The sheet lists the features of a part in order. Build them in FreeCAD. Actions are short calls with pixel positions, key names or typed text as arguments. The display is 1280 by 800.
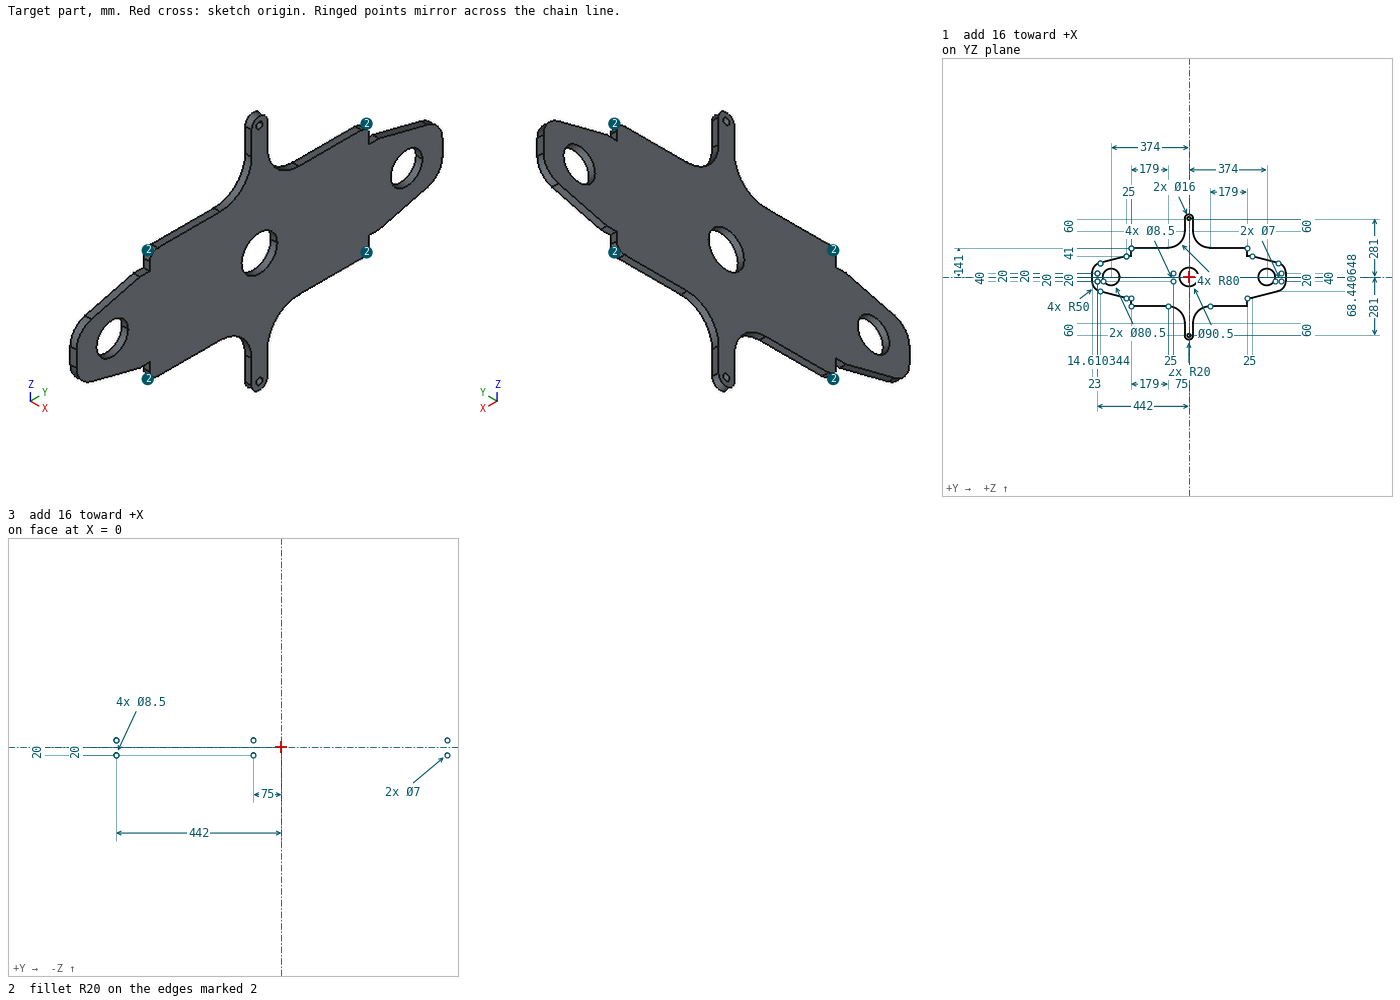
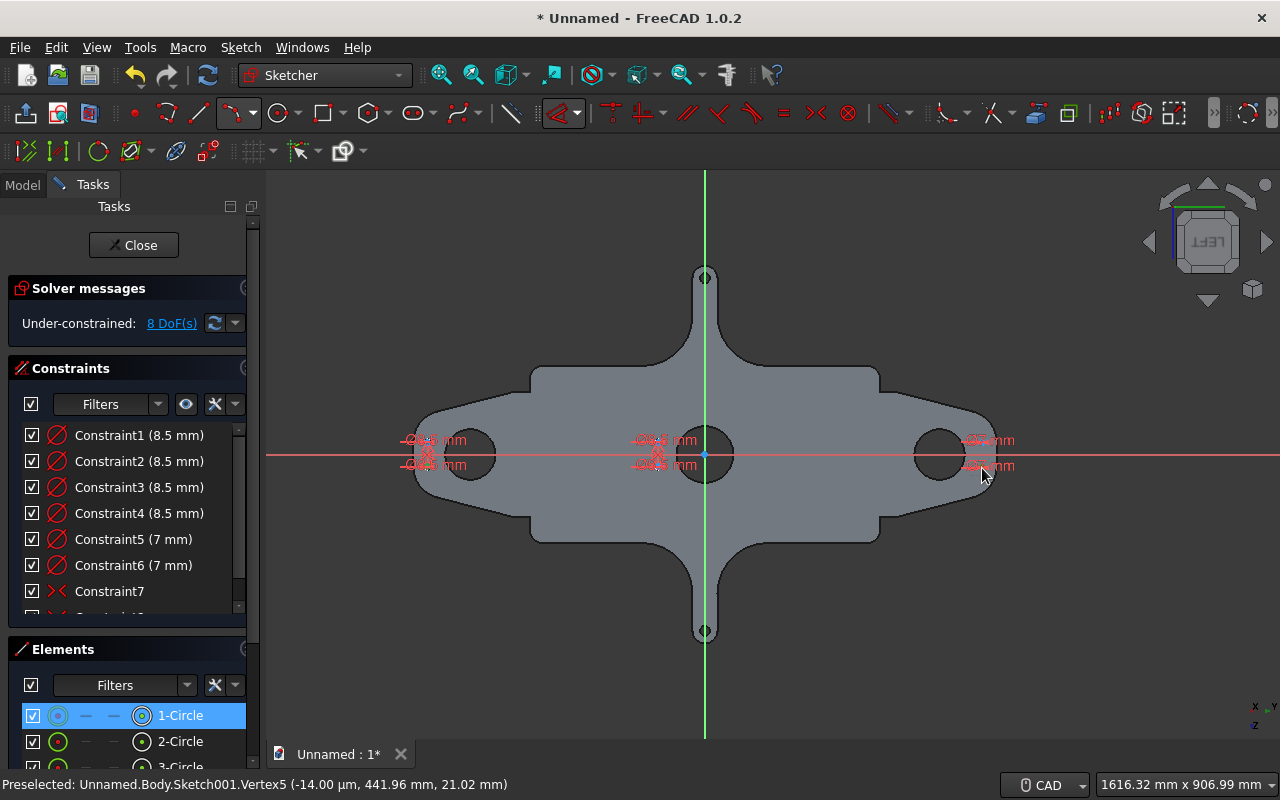
click(705, 674)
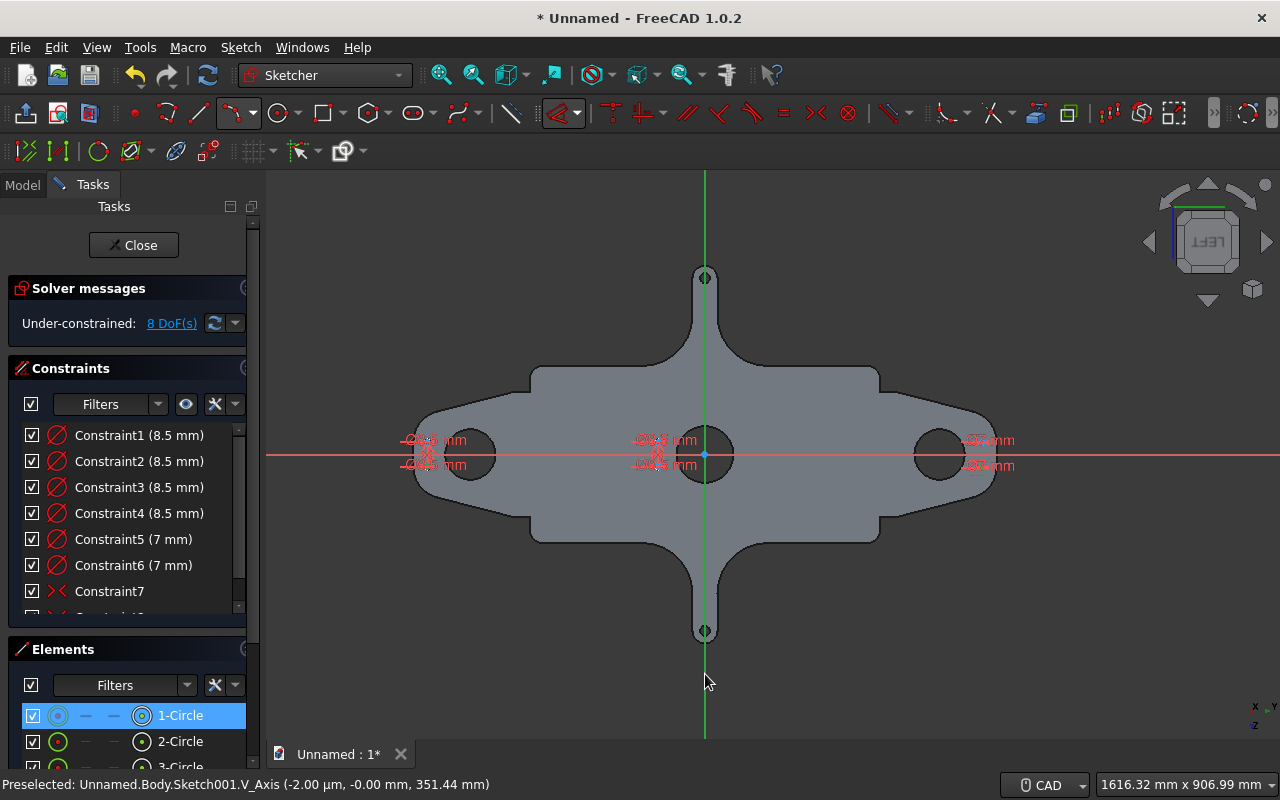
click(816, 114)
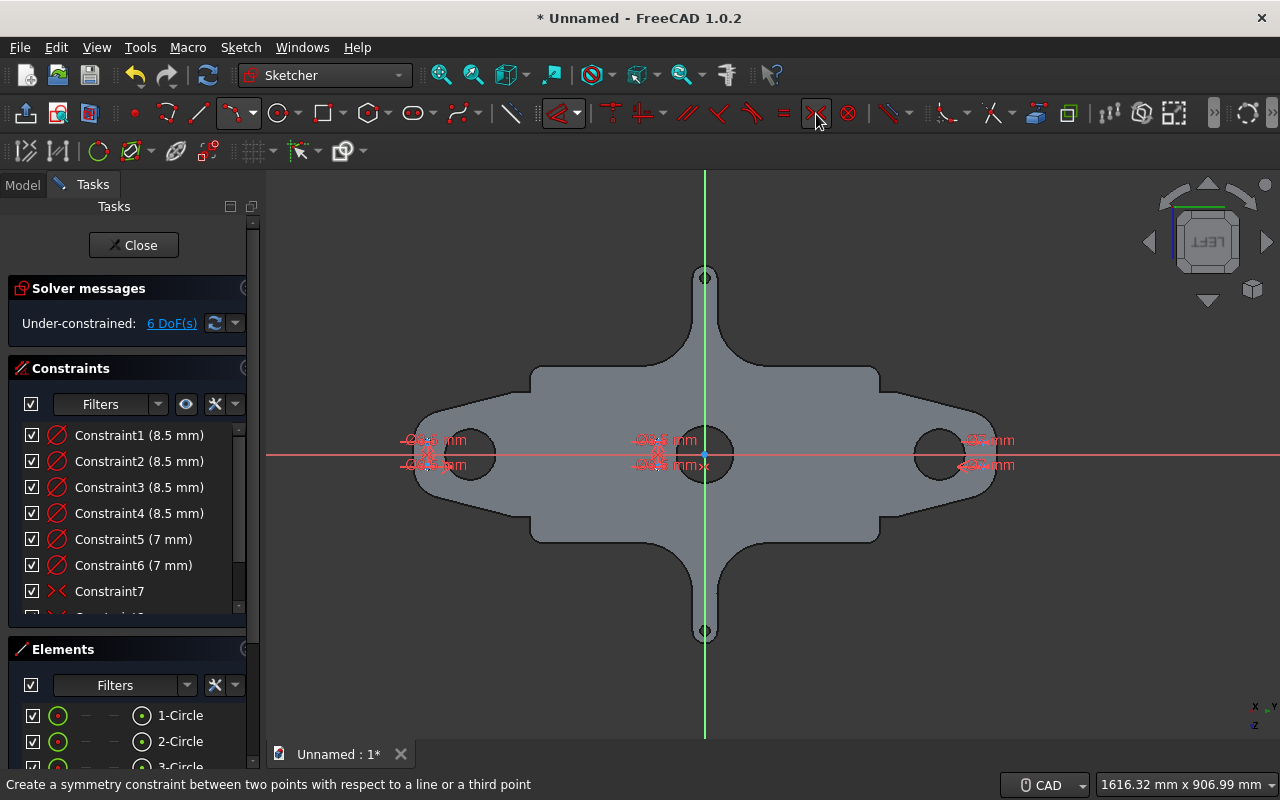
click(428, 442)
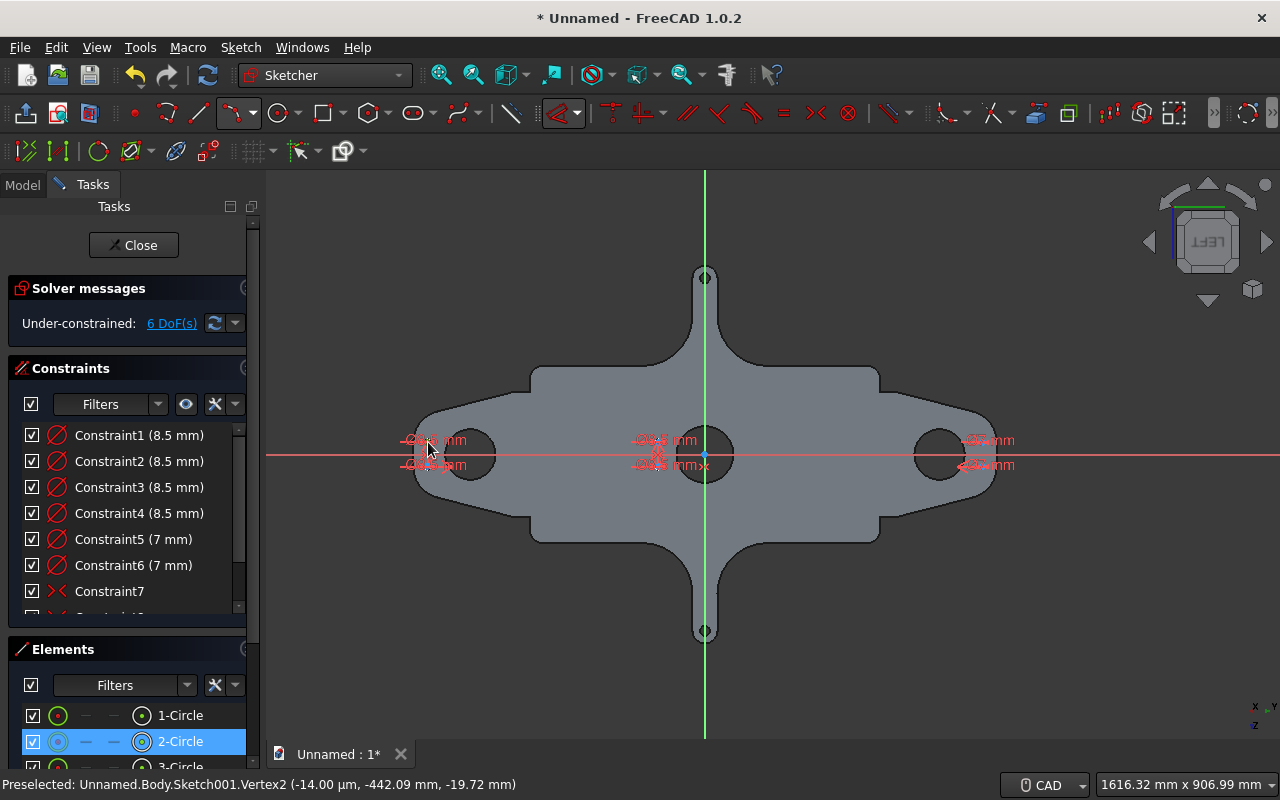
click(982, 442)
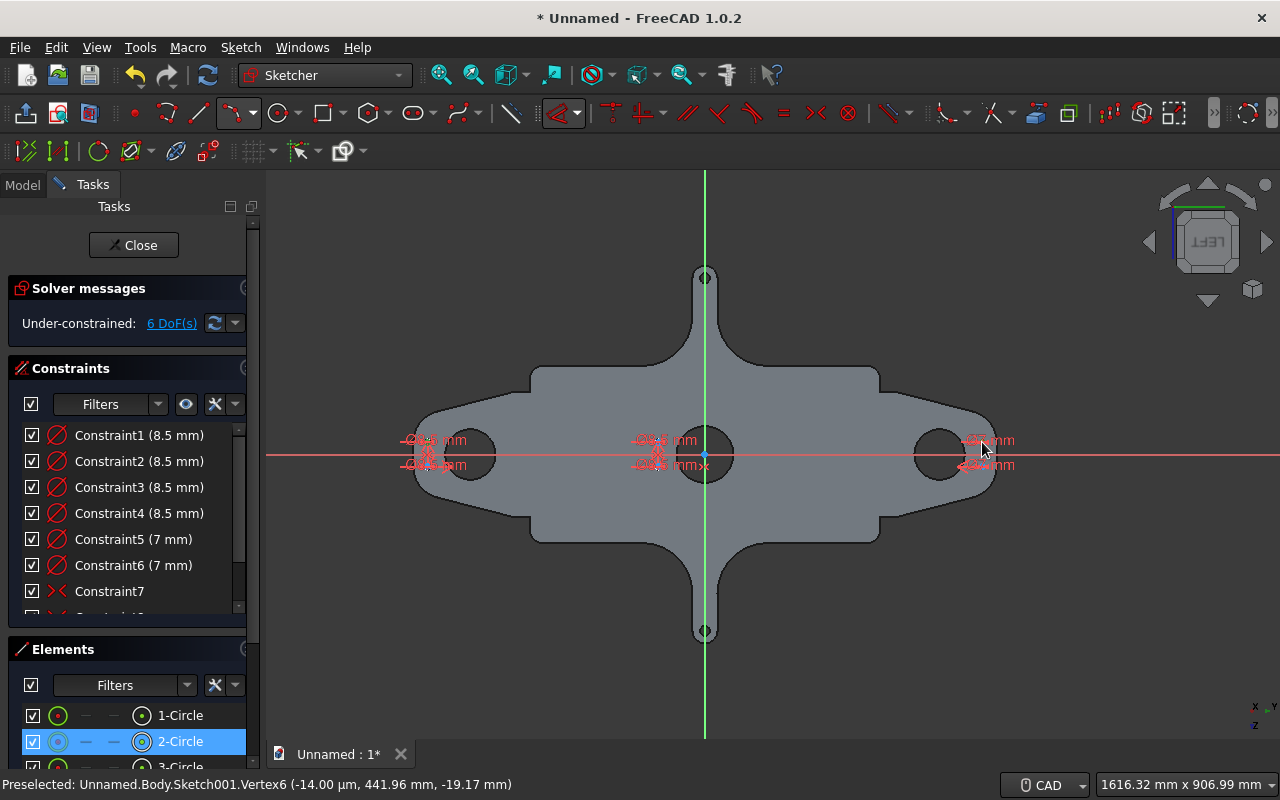
click(705, 674)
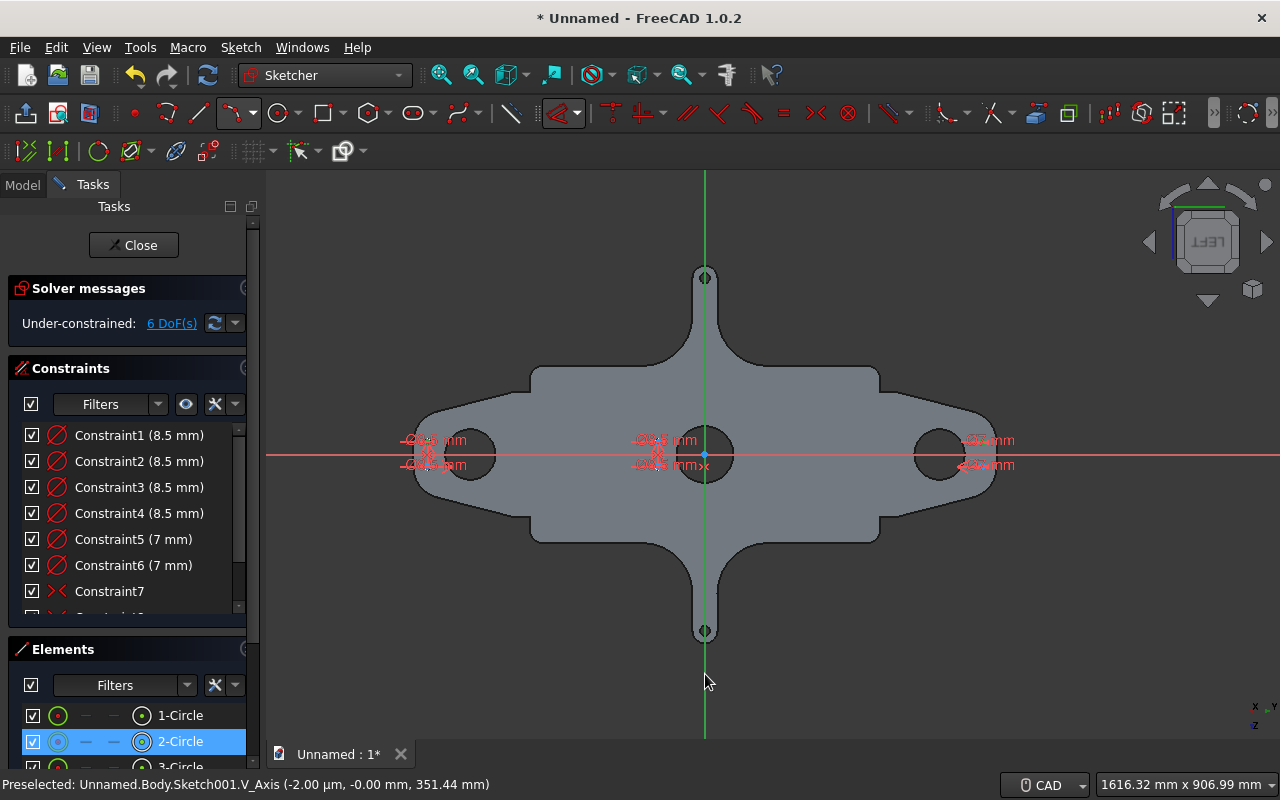
click(816, 114)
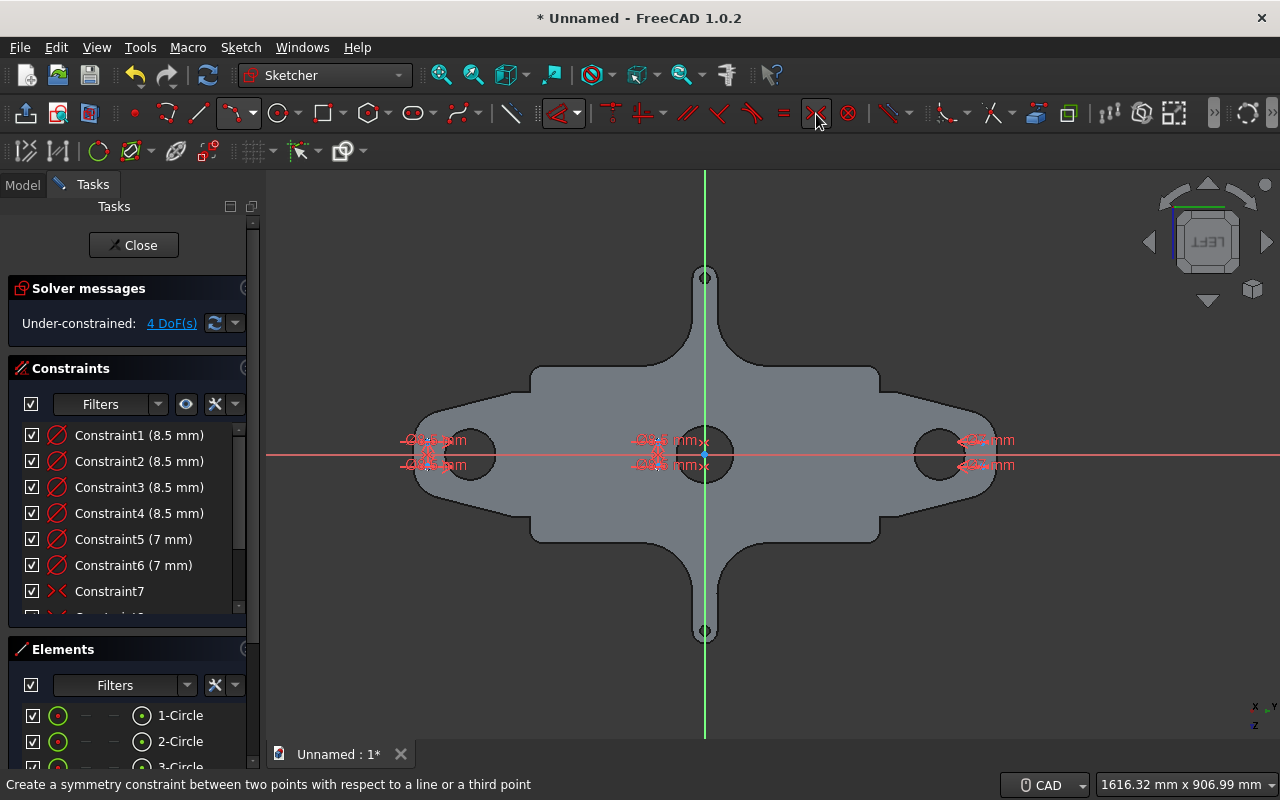
scroll(428, 467, up, 6)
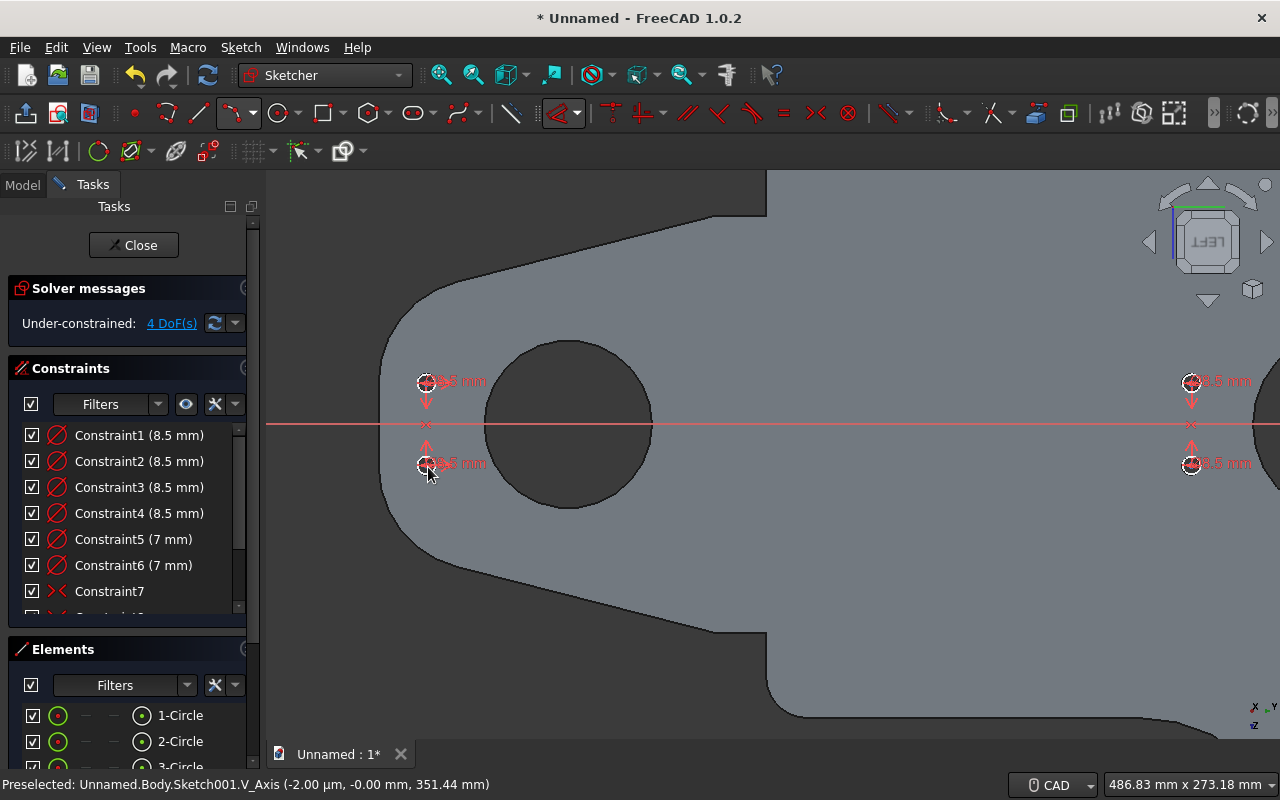
click(426, 465)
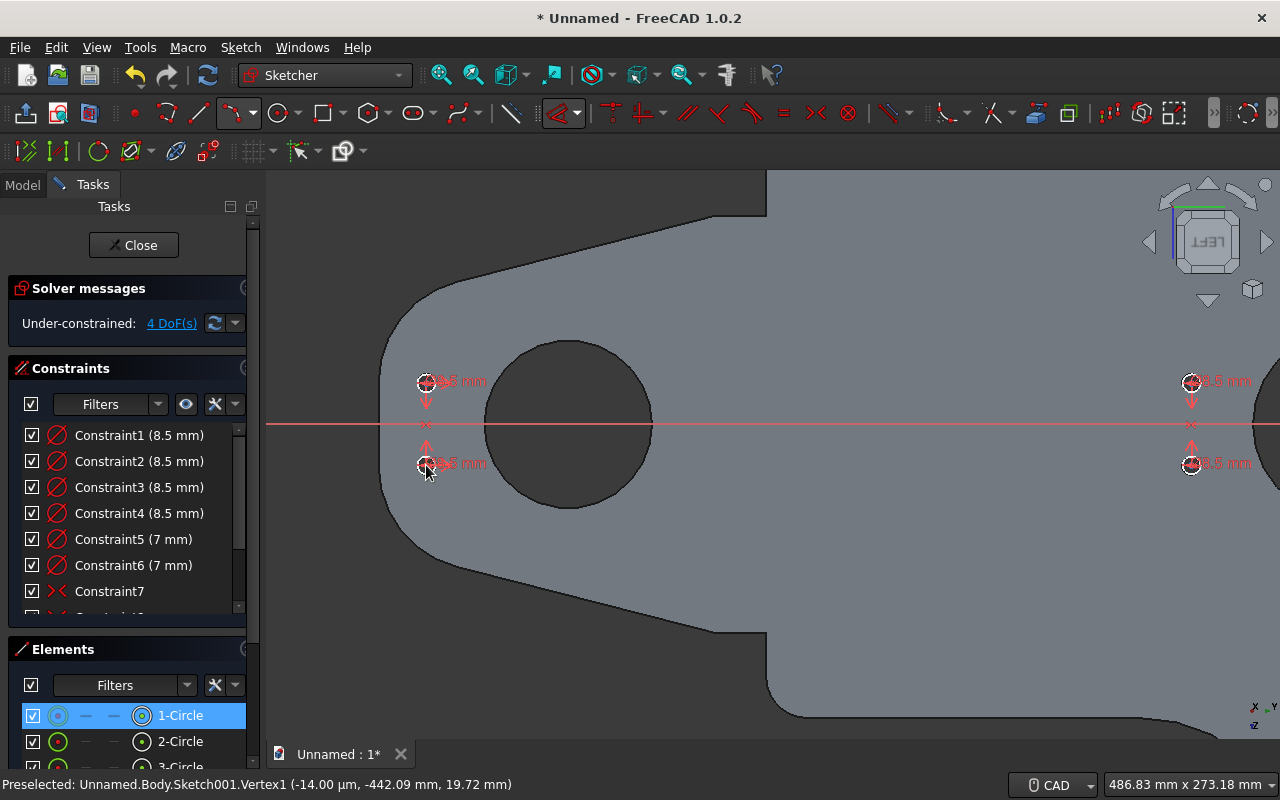
key(i)